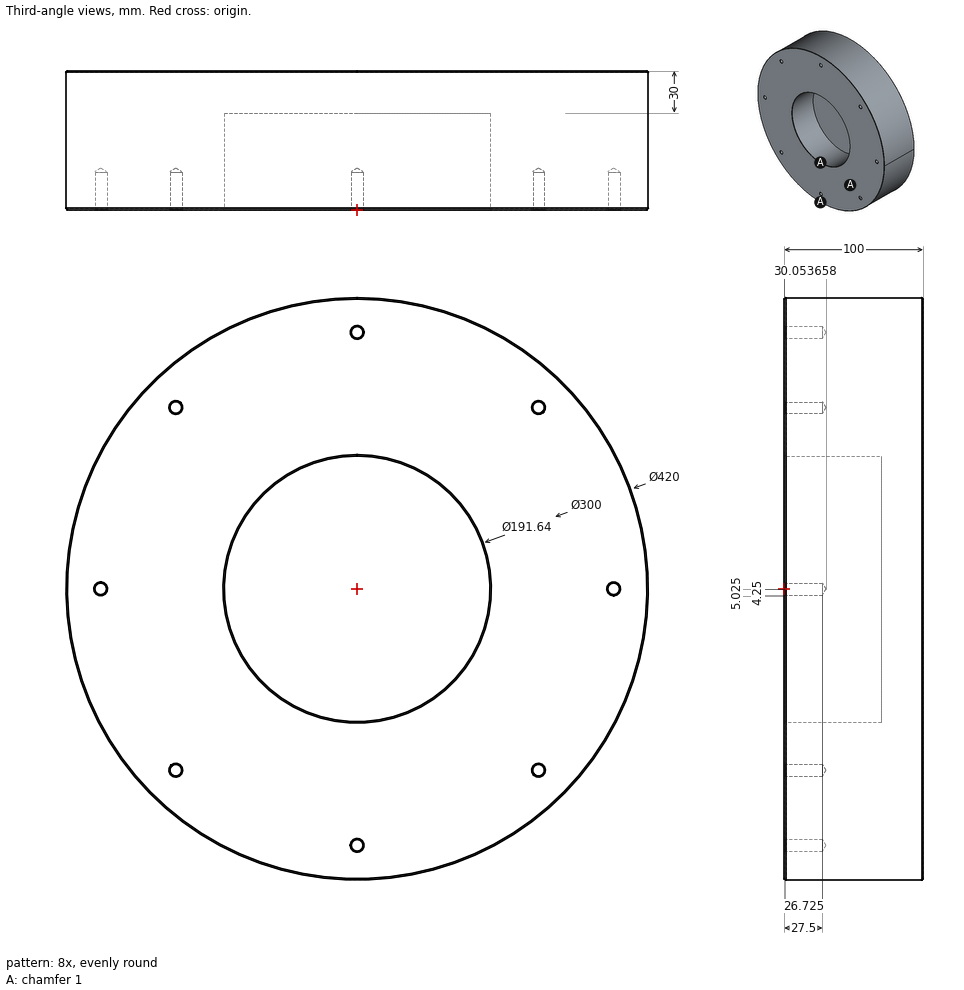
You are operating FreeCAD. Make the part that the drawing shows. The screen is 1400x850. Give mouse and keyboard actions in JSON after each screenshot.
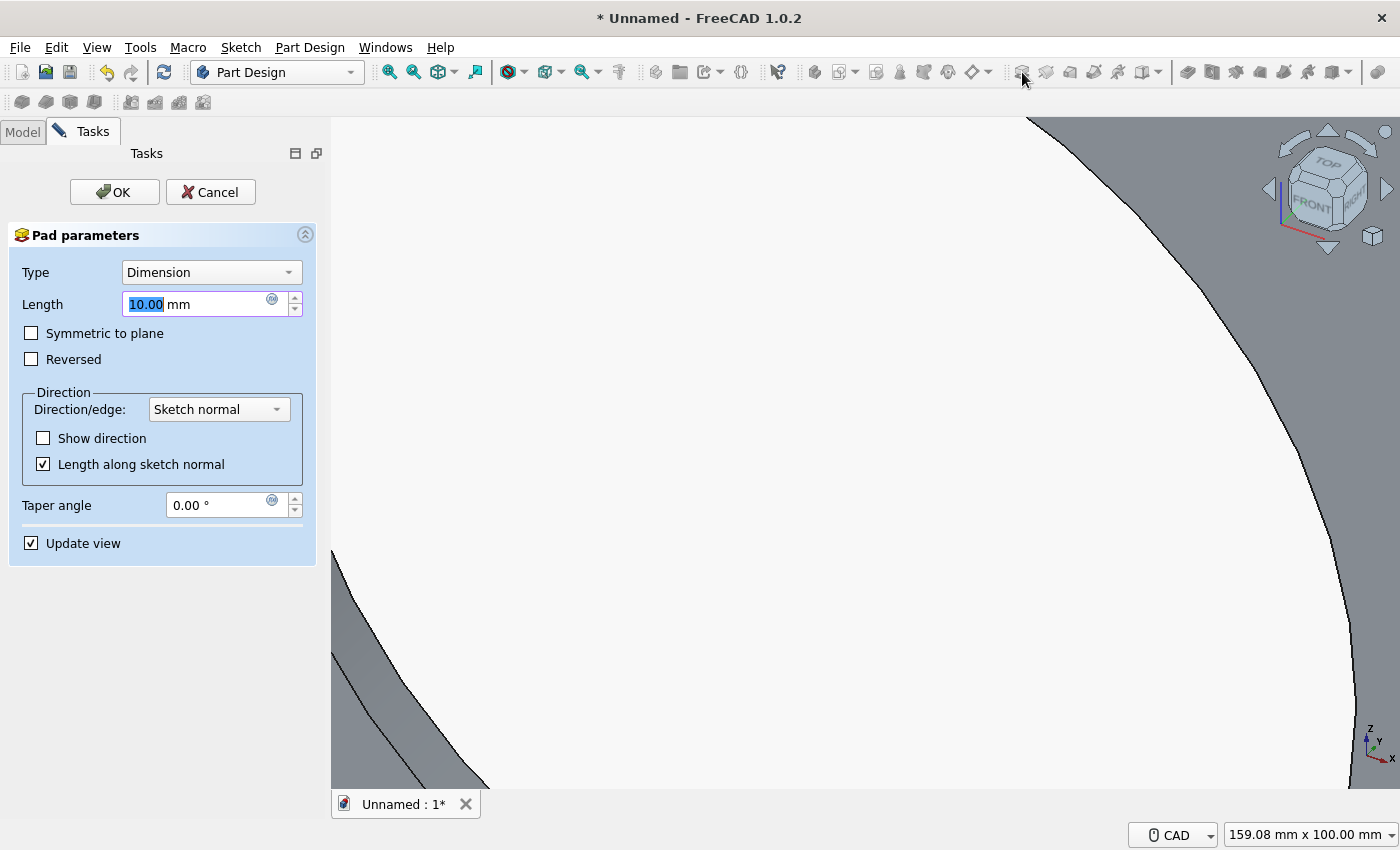
{"action": "type", "text": "100"}
{"action": "key", "text": "Tab"}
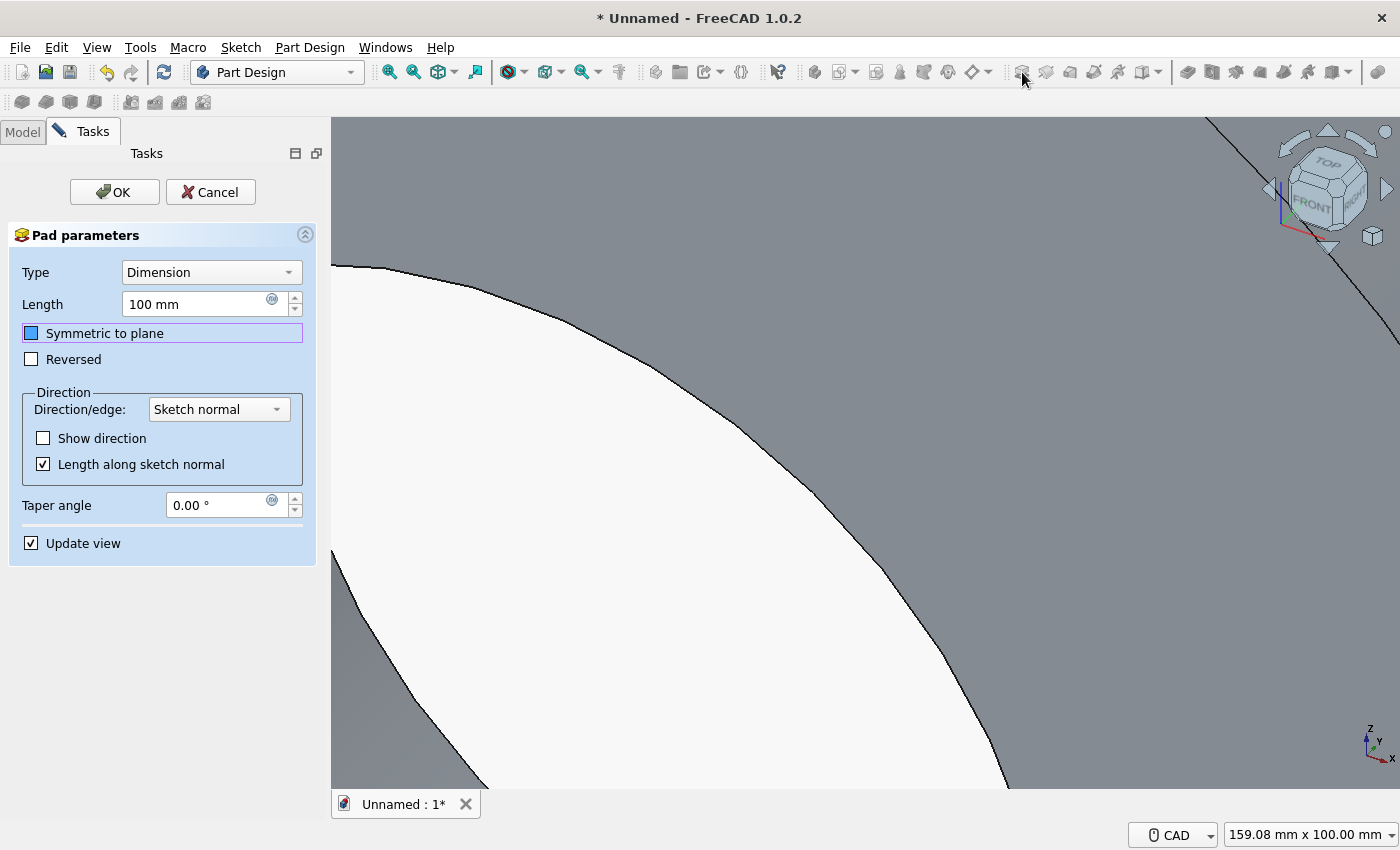
{"action": "left_click", "coordinate": [30, 359]}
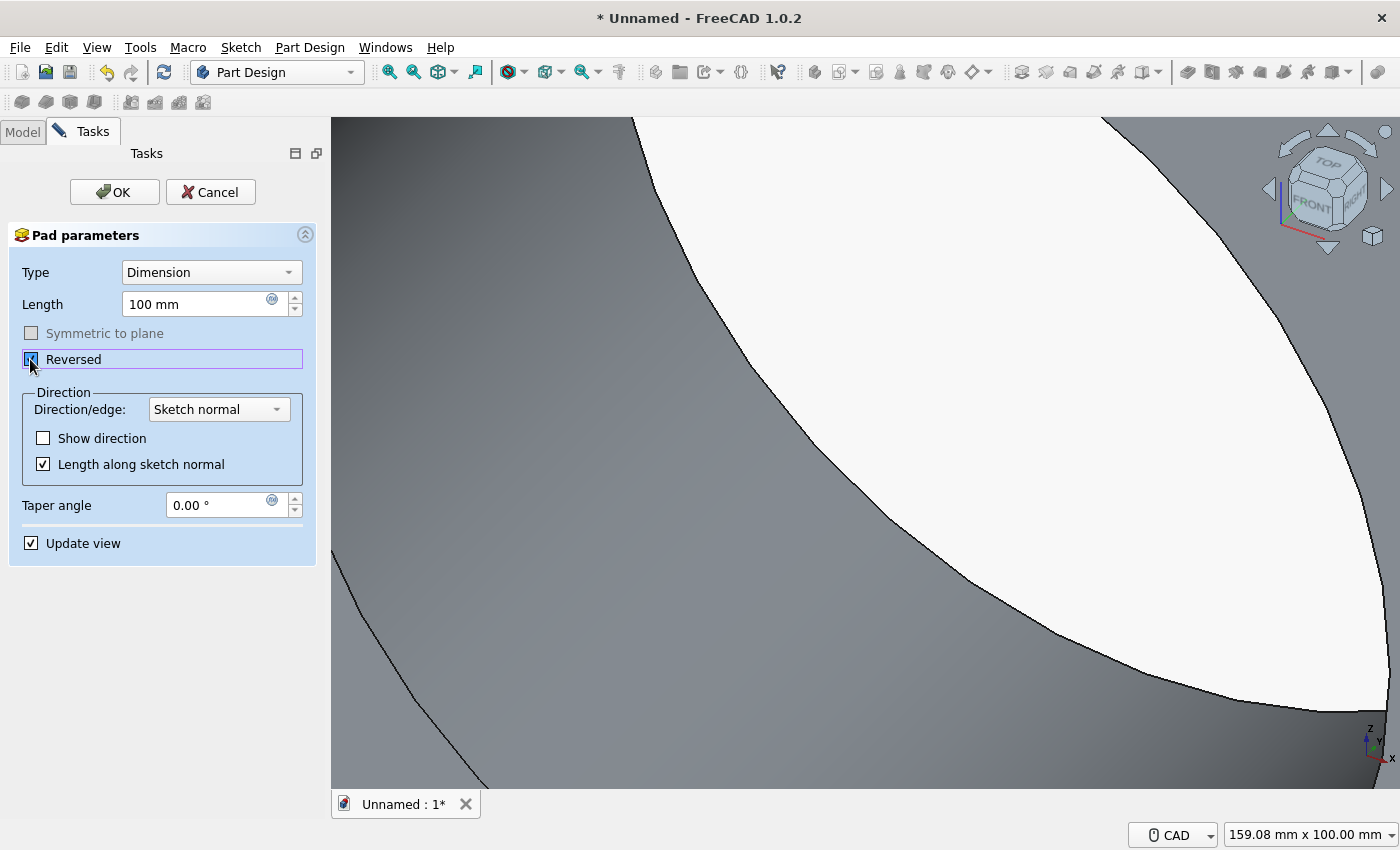
{"action": "left_click", "coordinate": [115, 192]}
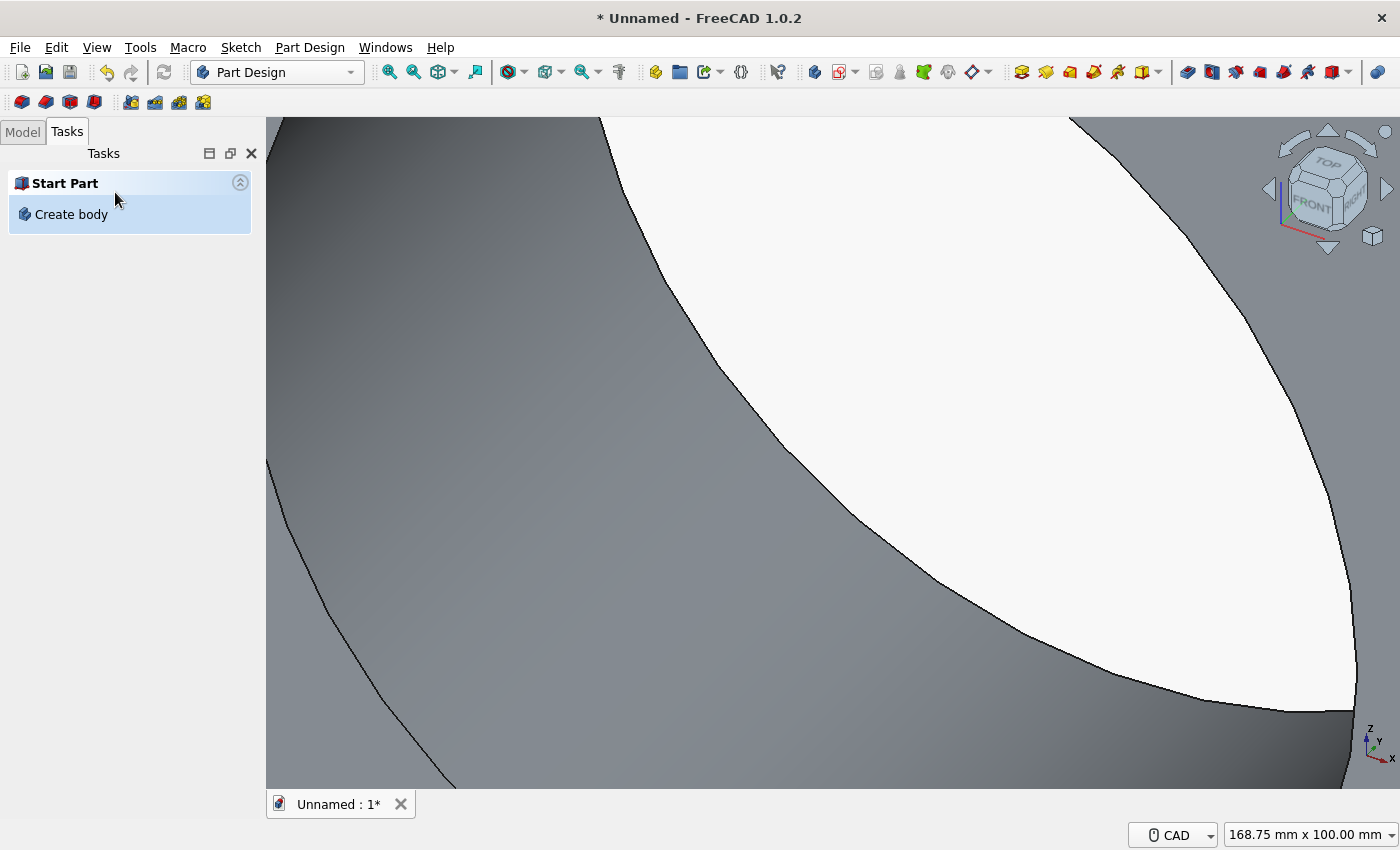
{"action": "key", "text": "v f"}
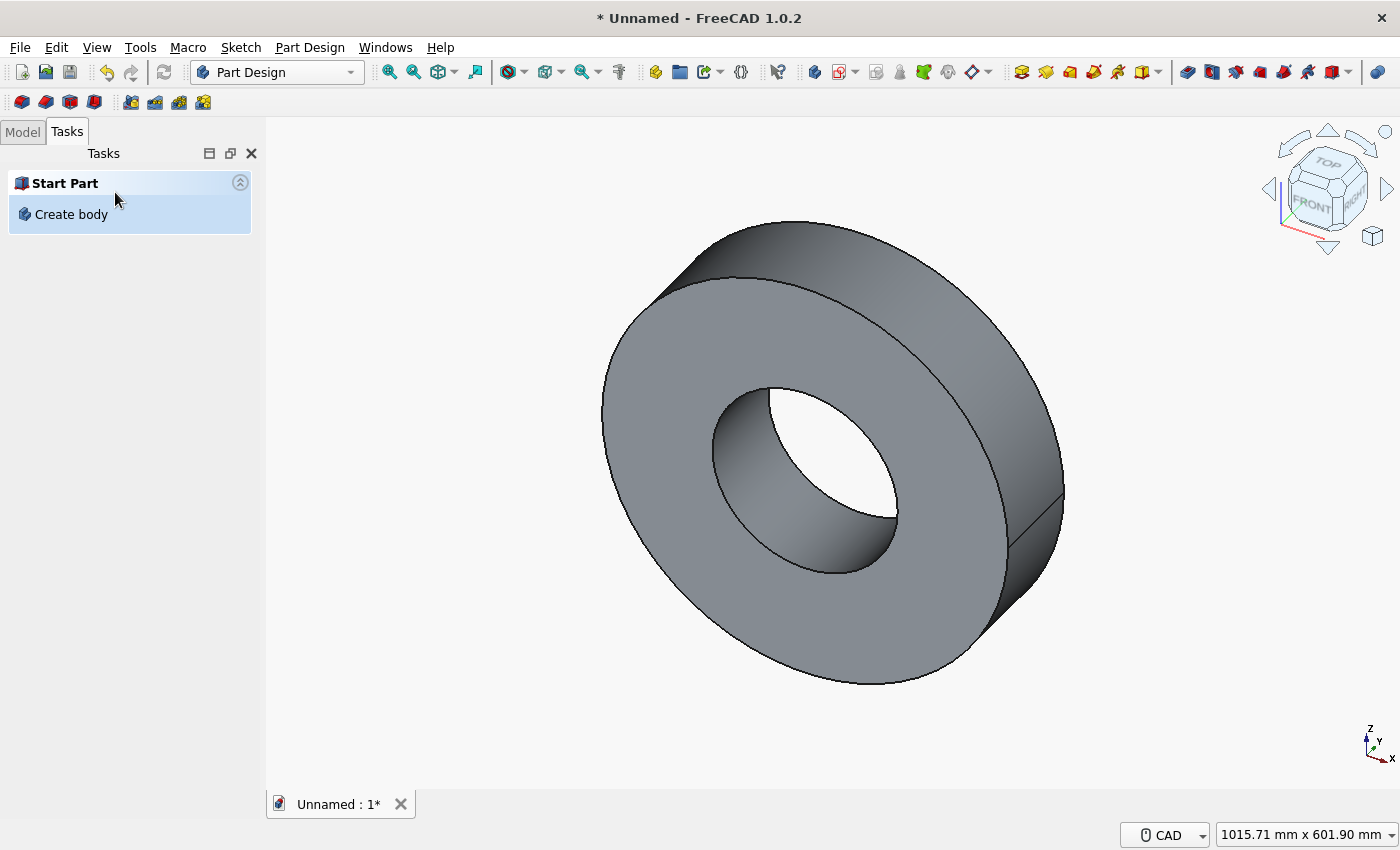
{"action": "key", "text": "4"}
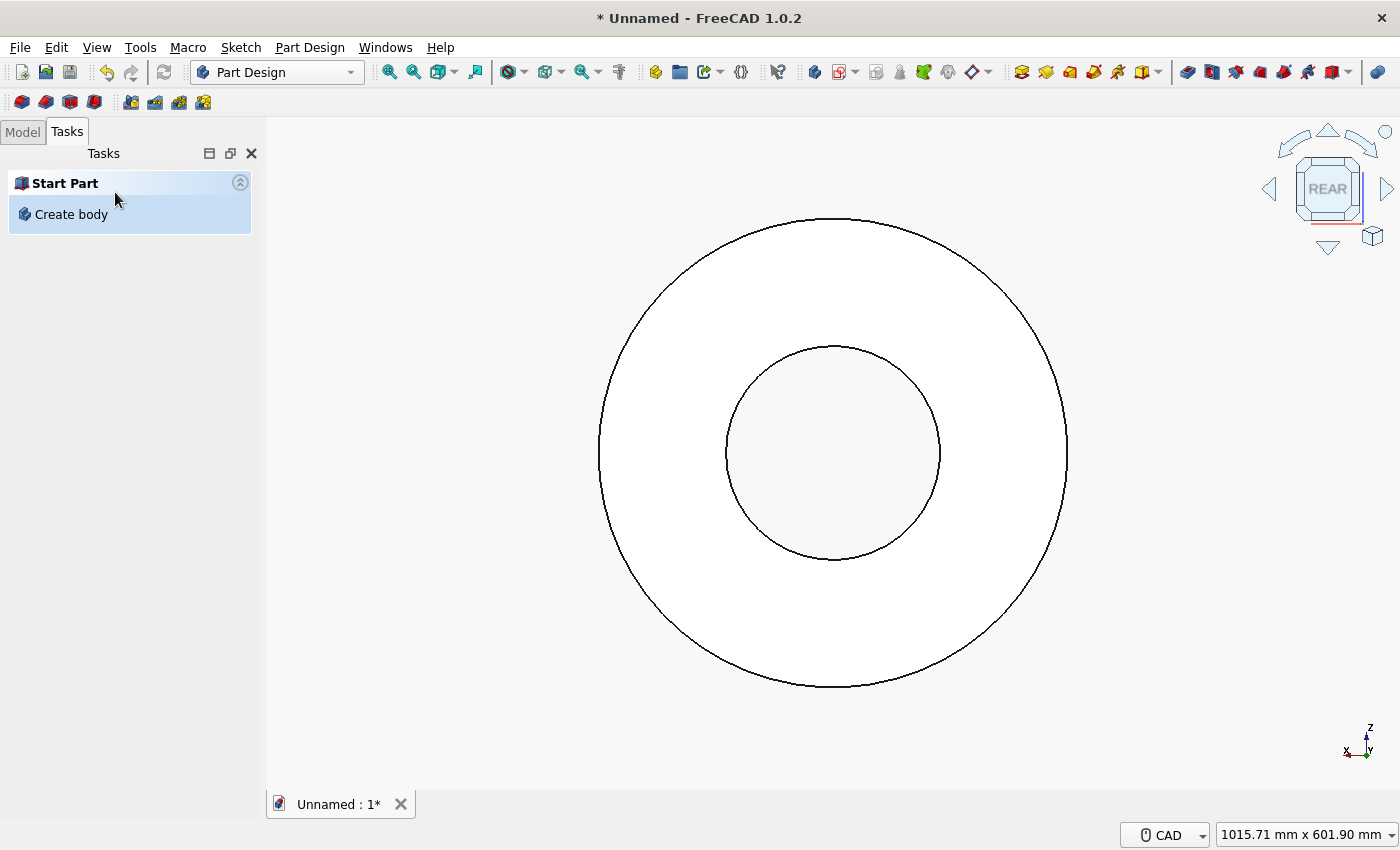
{"action": "left_click", "coordinate": [699, 318]}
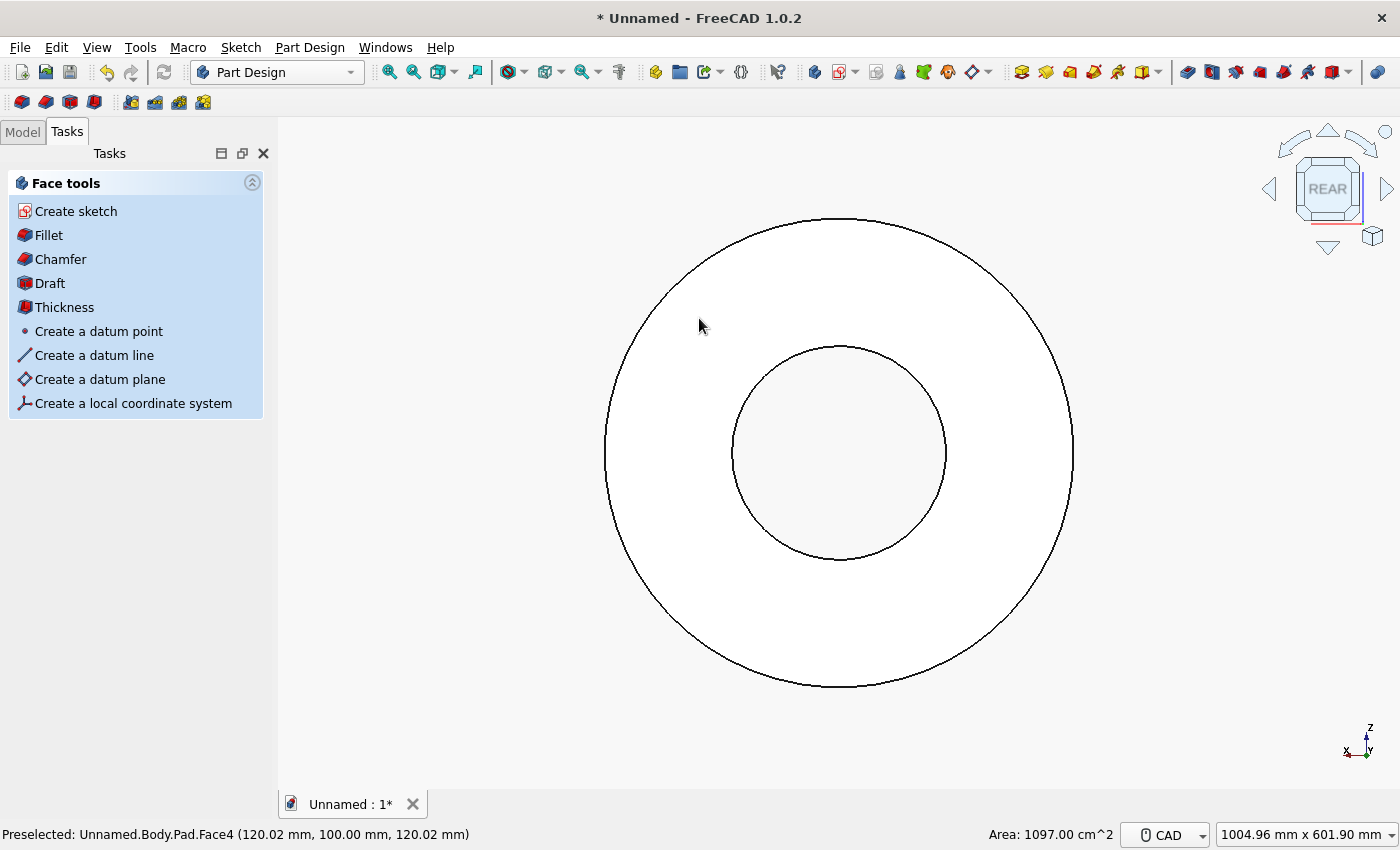
{"action": "left_click", "coordinate": [840, 72]}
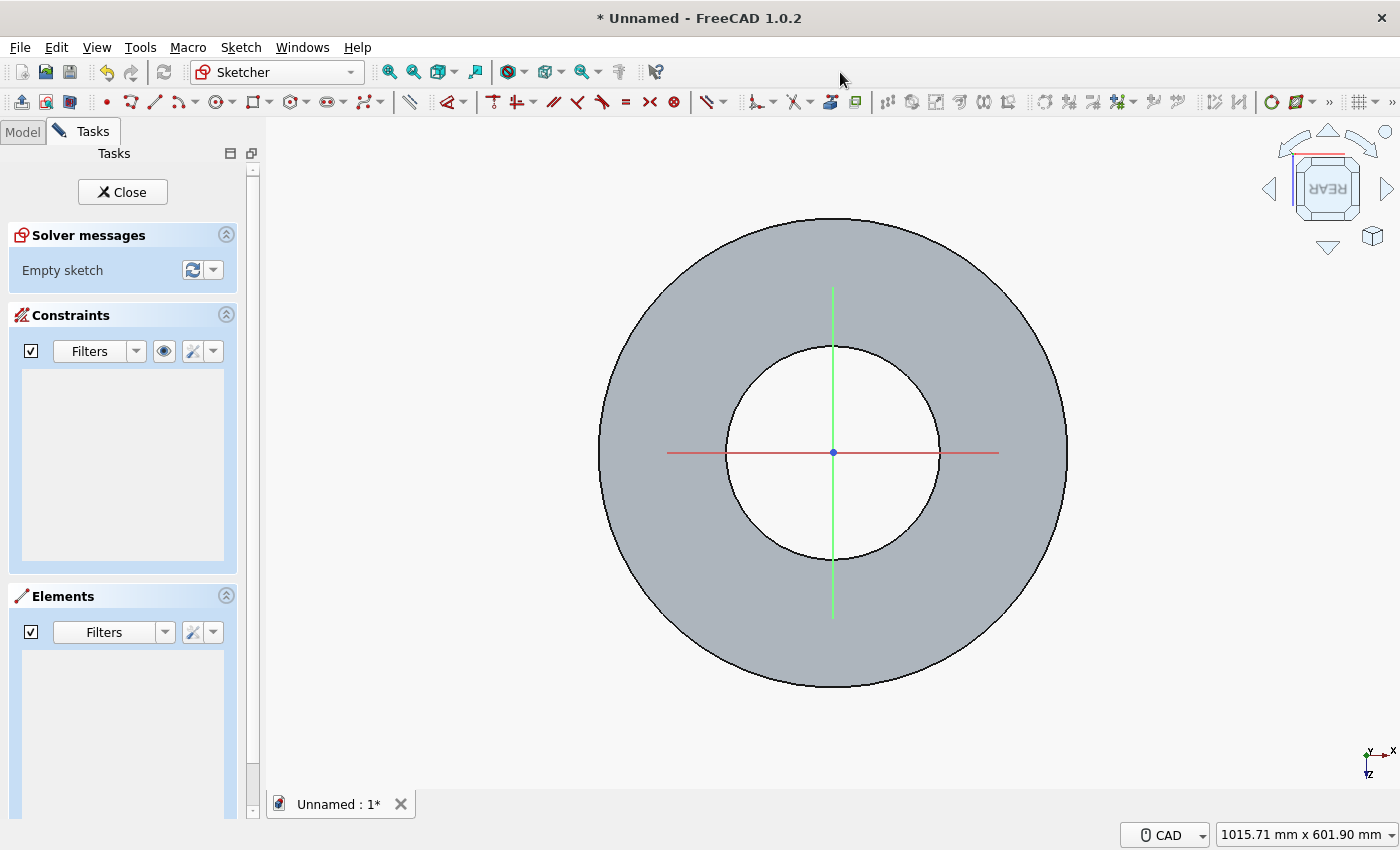
{"action": "key", "text": "g c"}